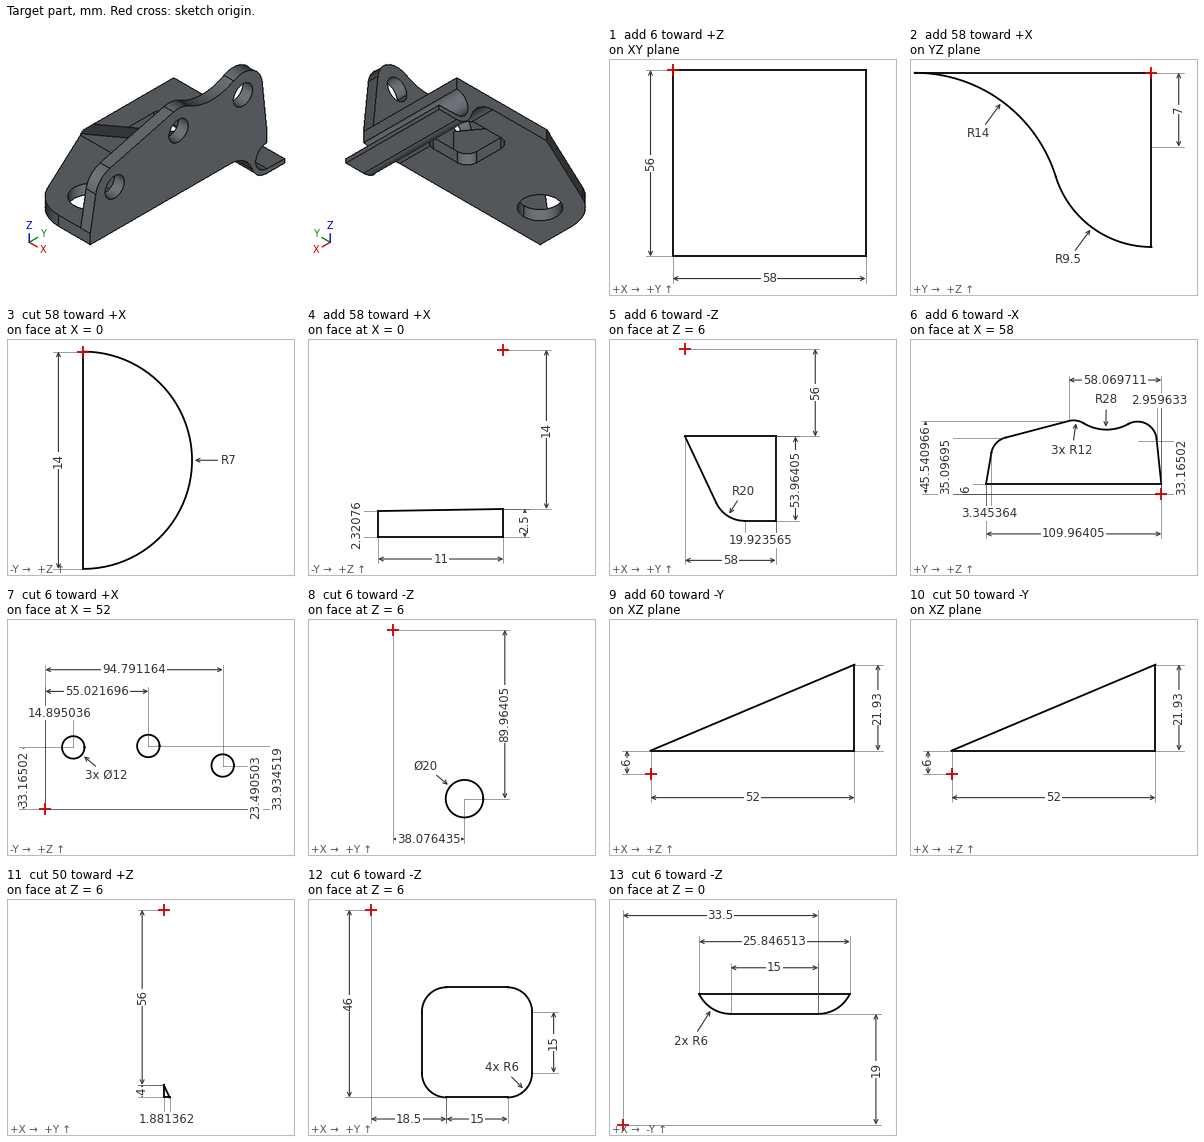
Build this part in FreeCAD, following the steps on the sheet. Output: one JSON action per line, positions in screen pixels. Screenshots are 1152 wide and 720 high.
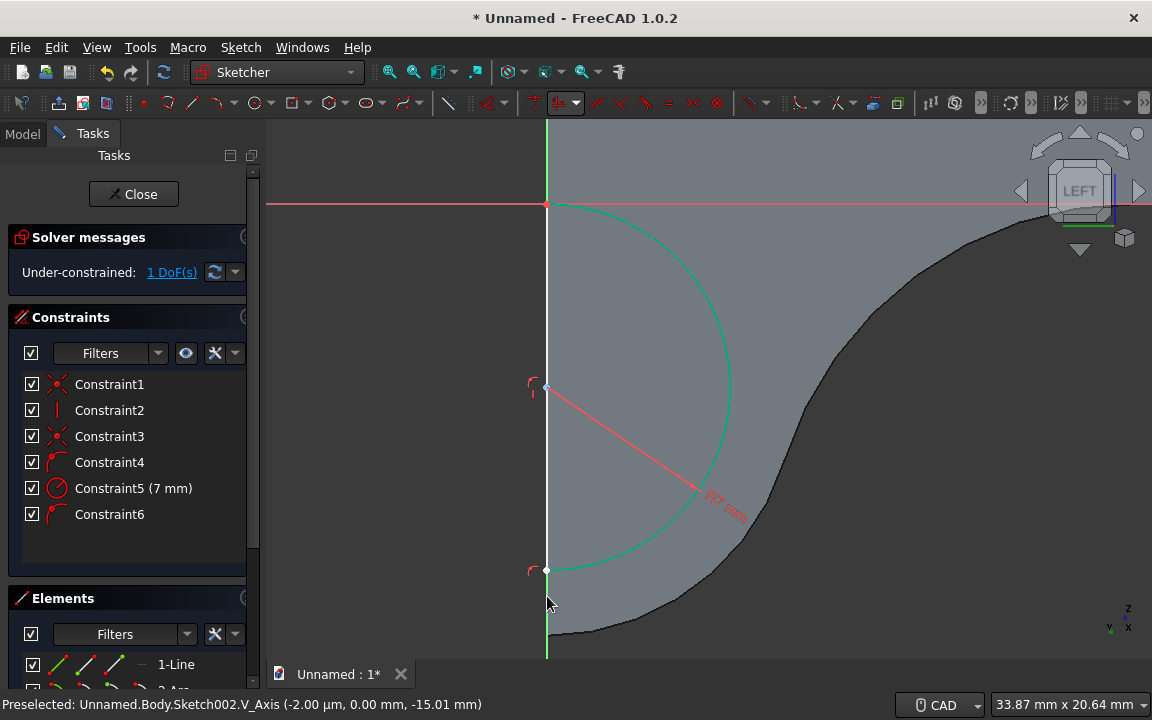
{"action": "key", "text": "d"}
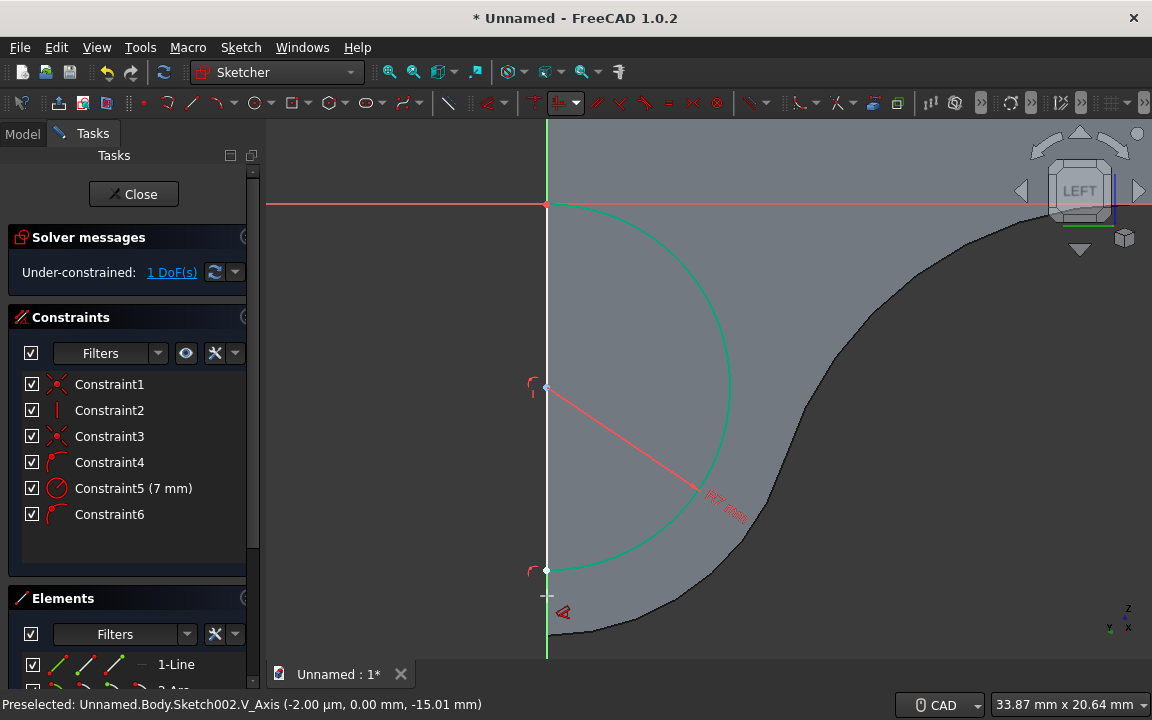
{"action": "left_click", "coordinate": [547, 314]}
{"action": "left_click", "coordinate": [513, 388]}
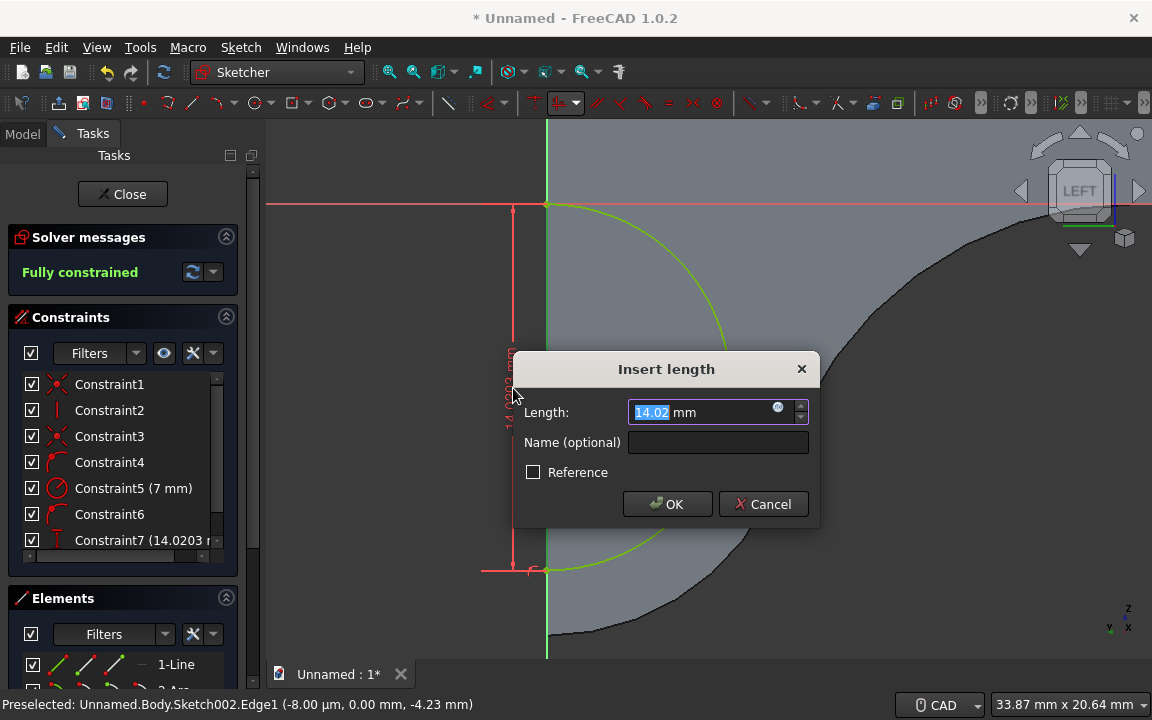
{"action": "type", "text": "14"}
{"action": "key", "text": "Return"}
{"action": "key", "text": "Escape"}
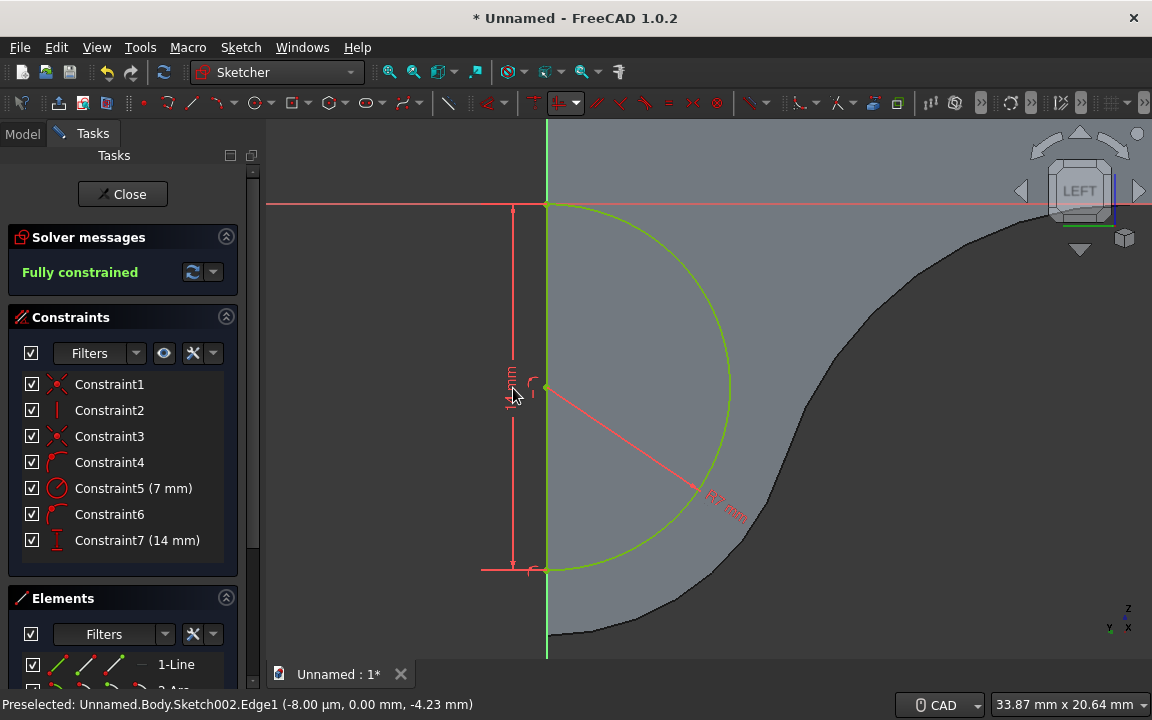
{"action": "left_click", "coordinate": [123, 194]}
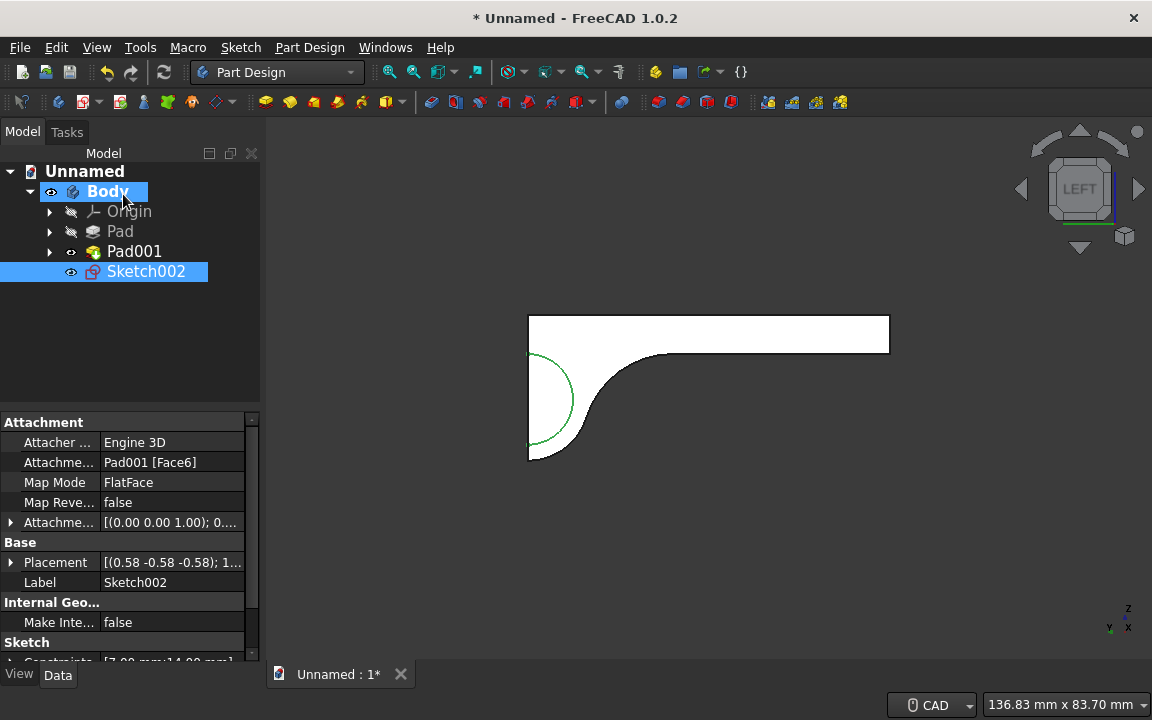
{"action": "left_click", "coordinate": [432, 102]}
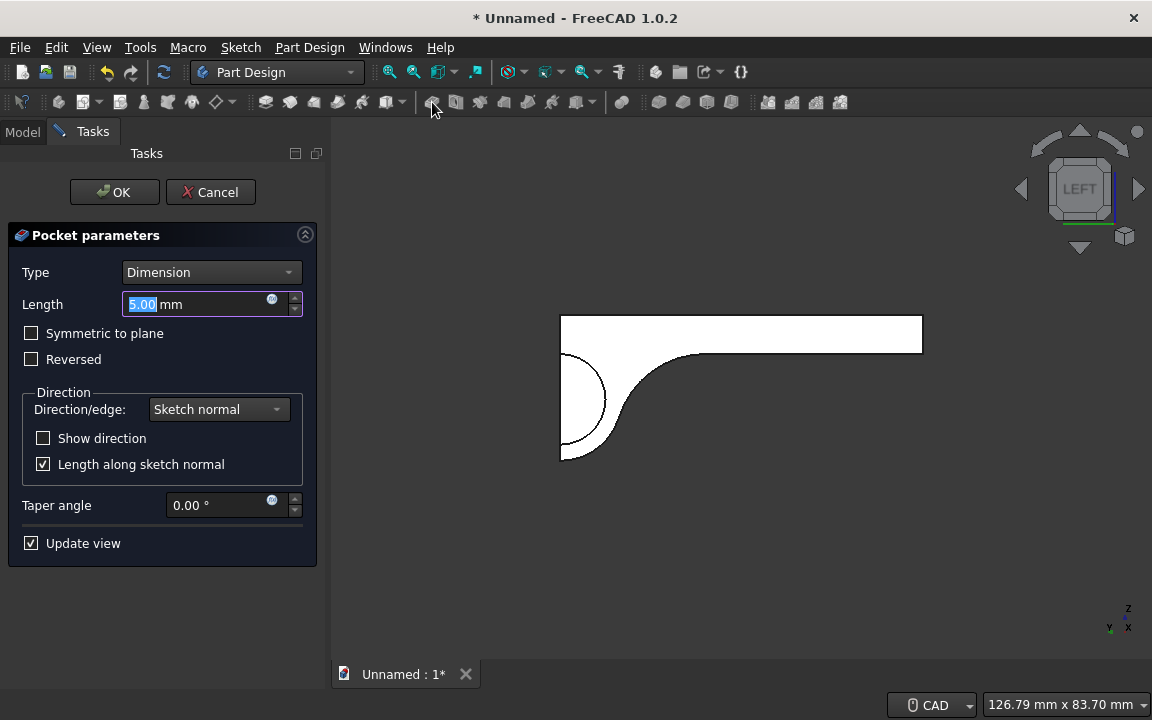
{"action": "type", "text": "58"}
{"action": "key", "text": "Tab"}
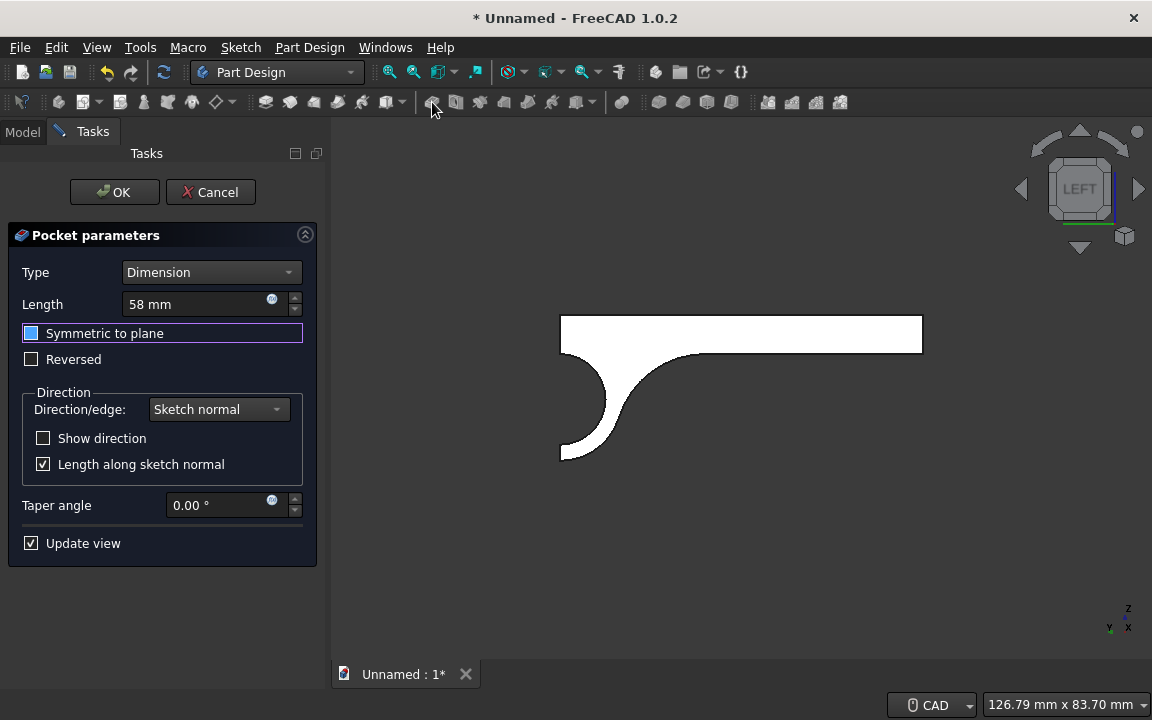
{"action": "left_click", "coordinate": [115, 192]}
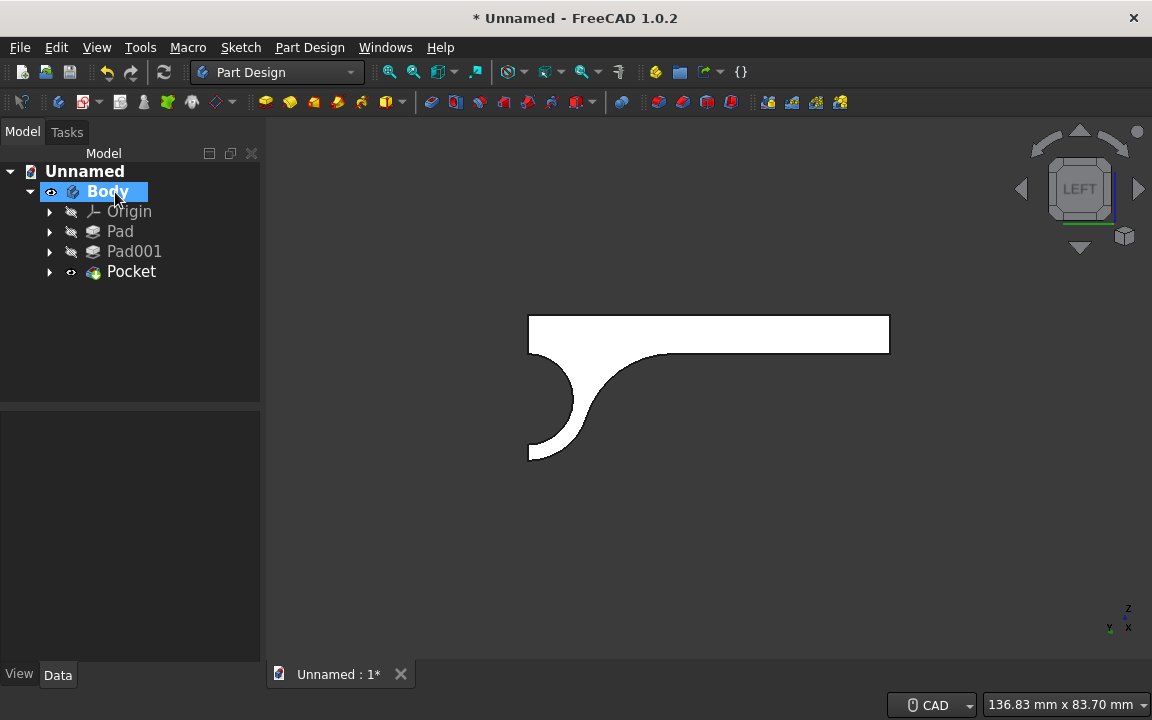
{"action": "left_click", "coordinate": [390, 72]}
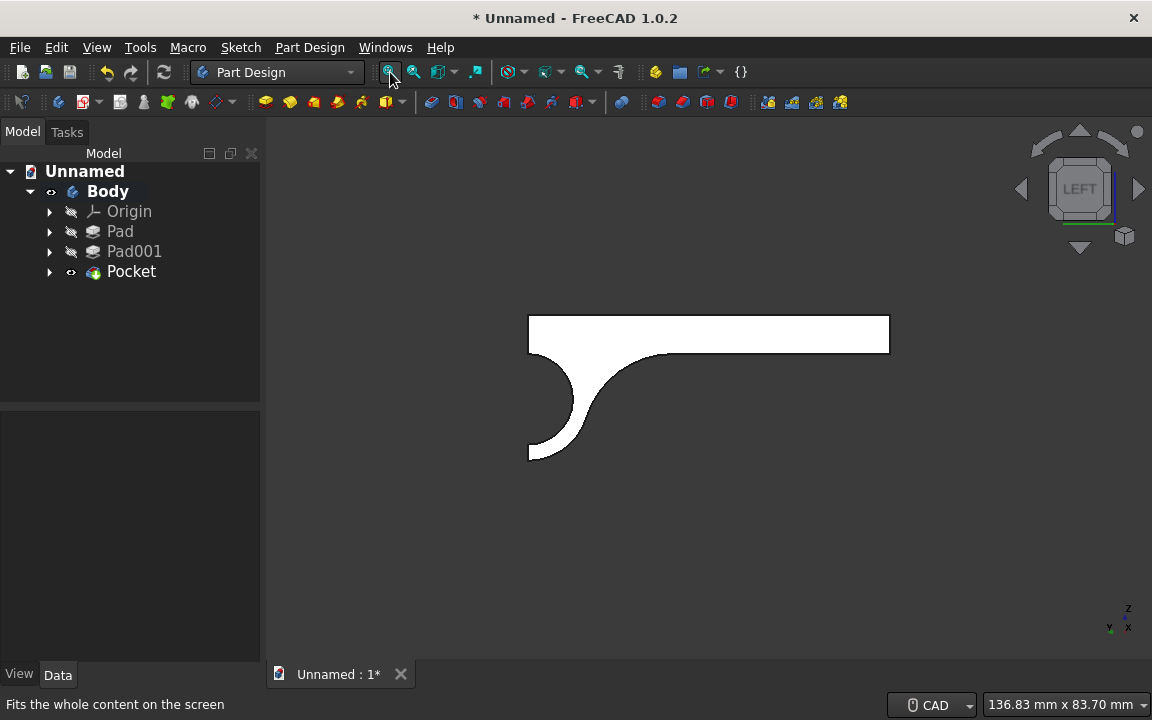
{"action": "left_click", "coordinate": [605, 345]}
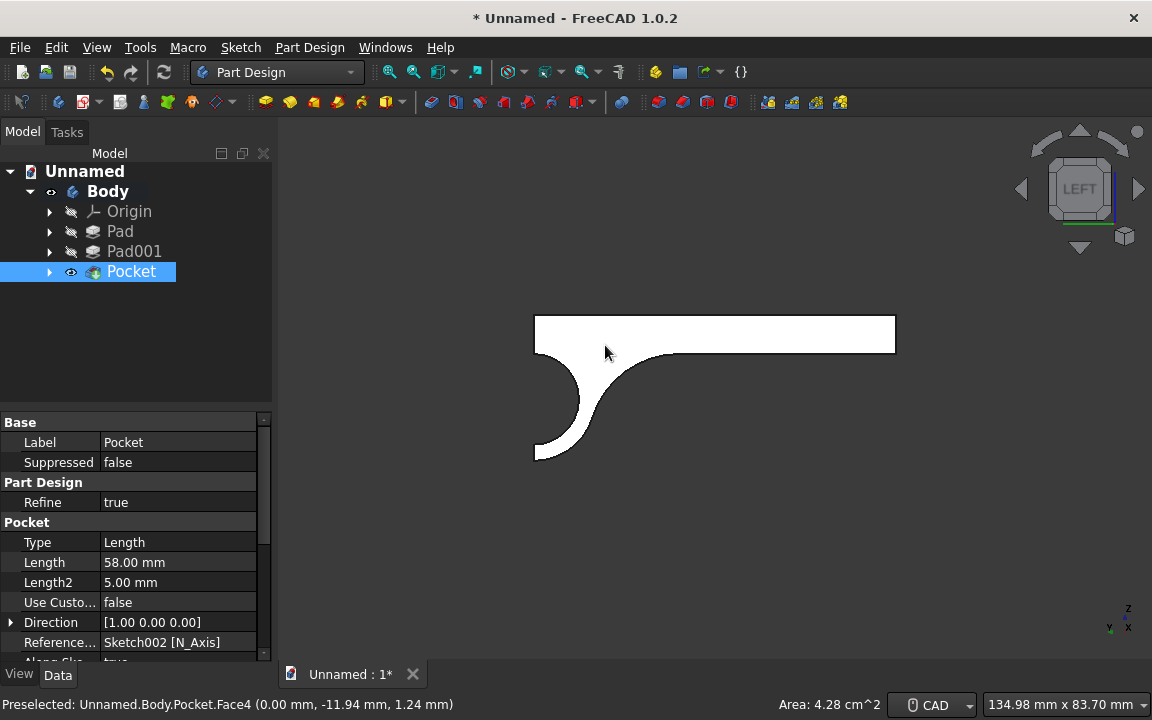
{"action": "left_click", "coordinate": [84, 102]}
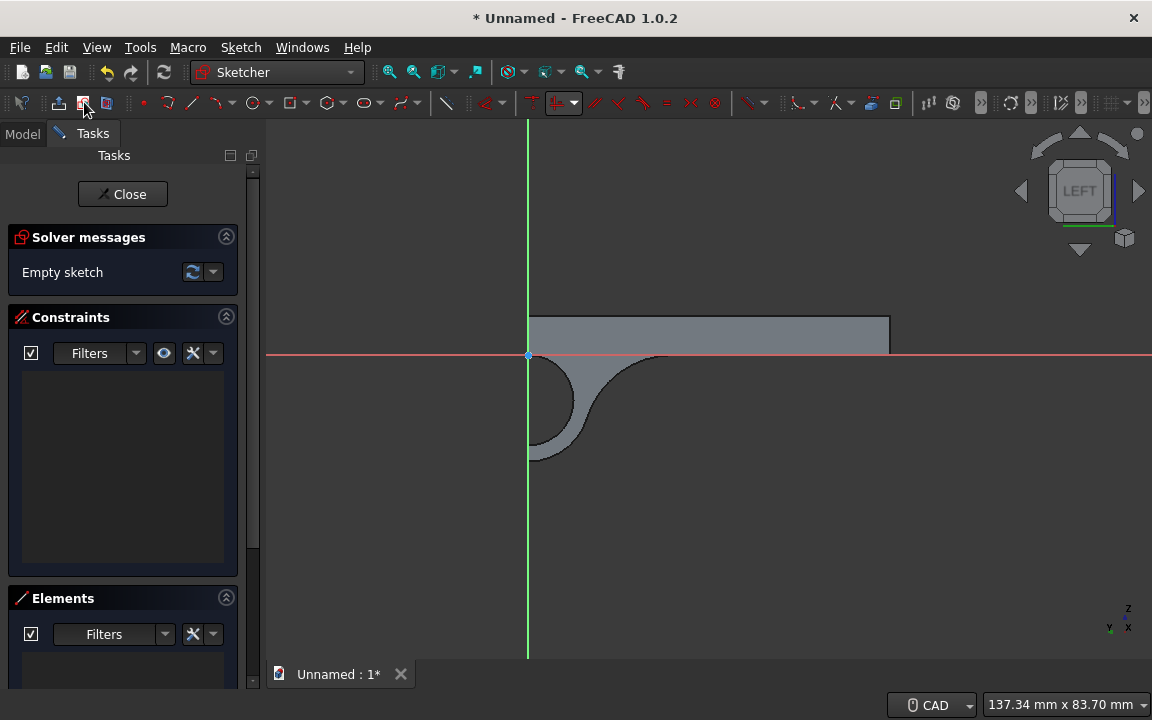
{"action": "scroll", "coordinate": [429, 417], "scroll_direction": "up", "scroll_amount": 6}